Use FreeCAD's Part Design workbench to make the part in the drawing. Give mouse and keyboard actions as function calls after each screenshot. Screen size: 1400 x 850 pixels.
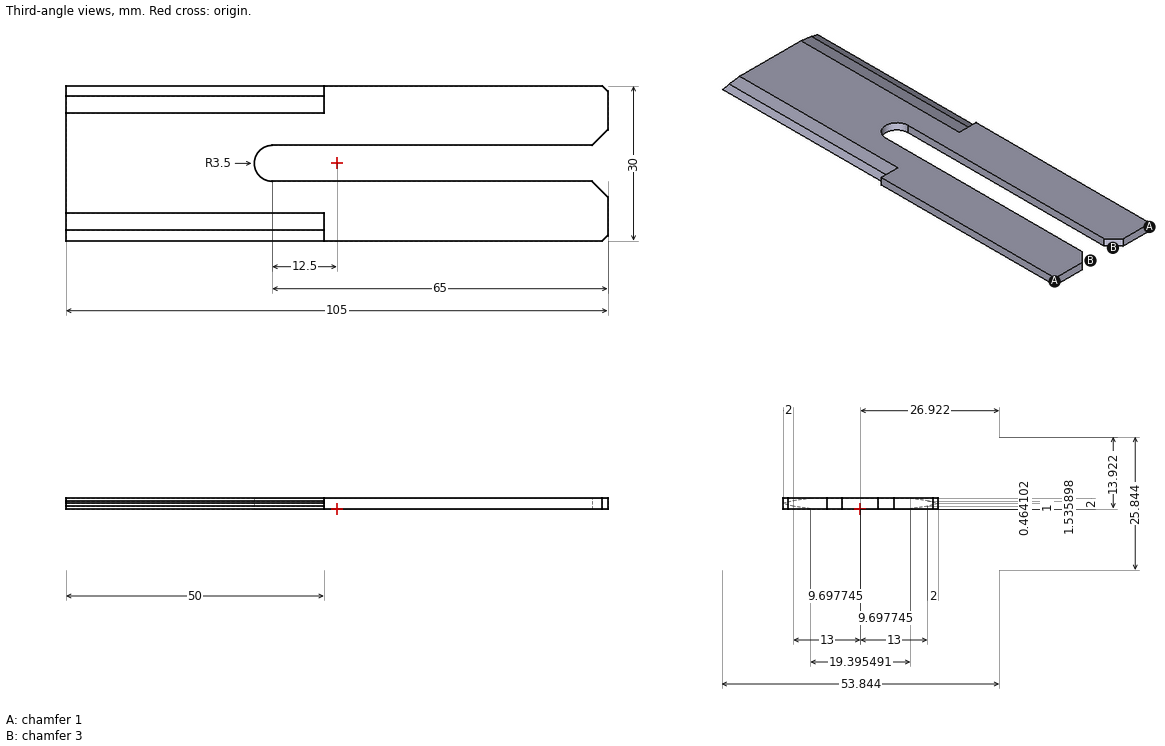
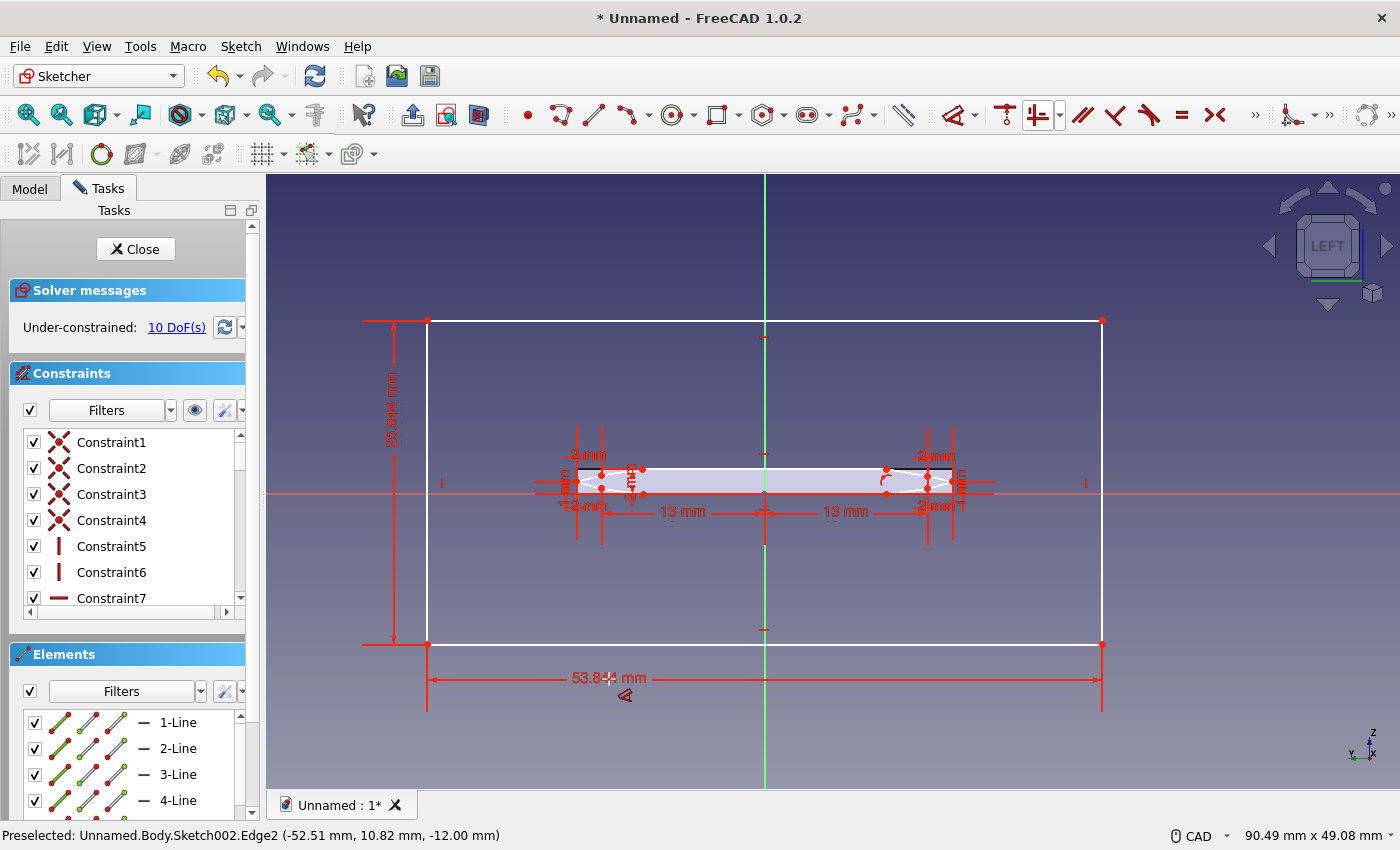
click(427, 321)
click(596, 287)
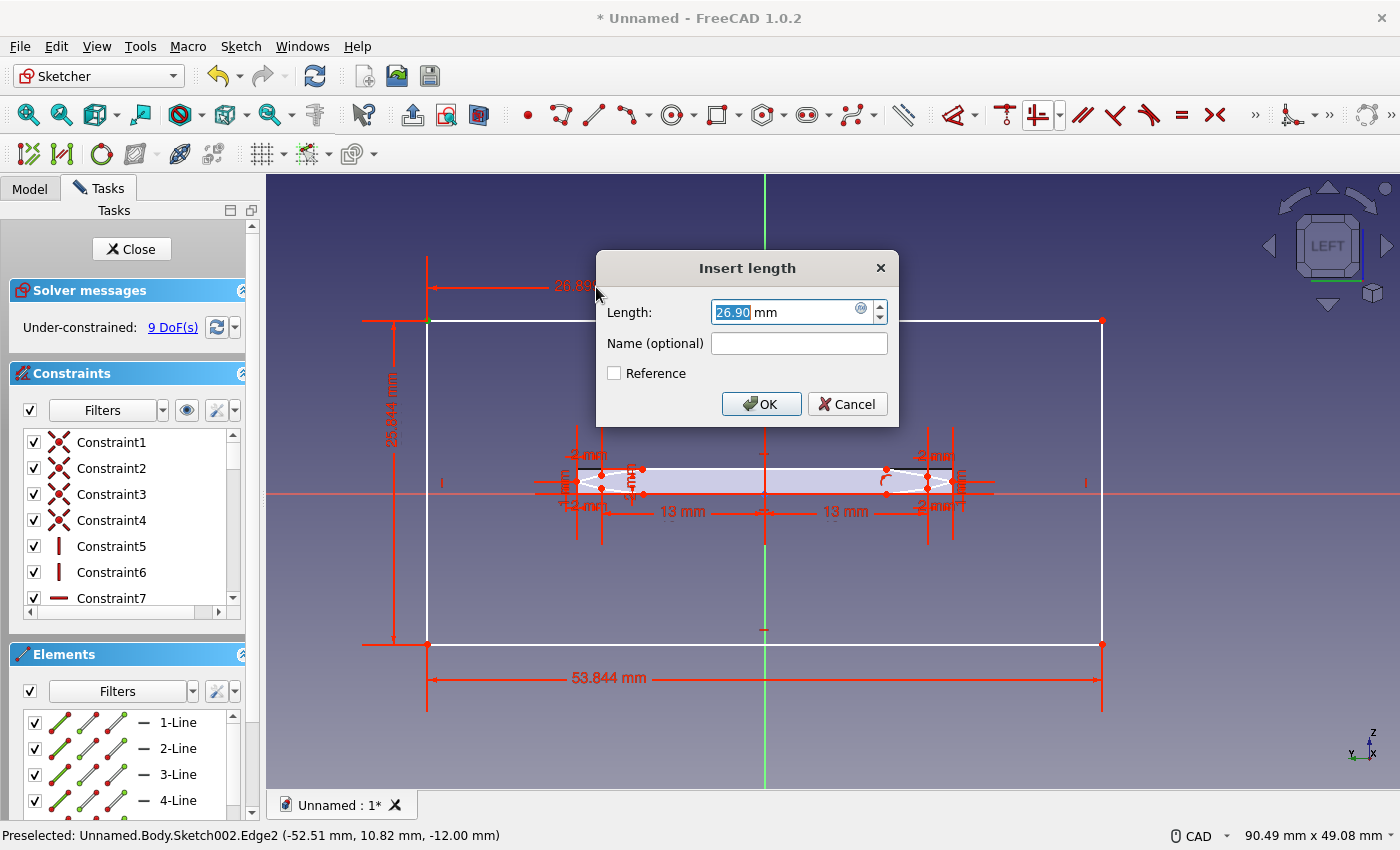
text(26.922)
key(Return)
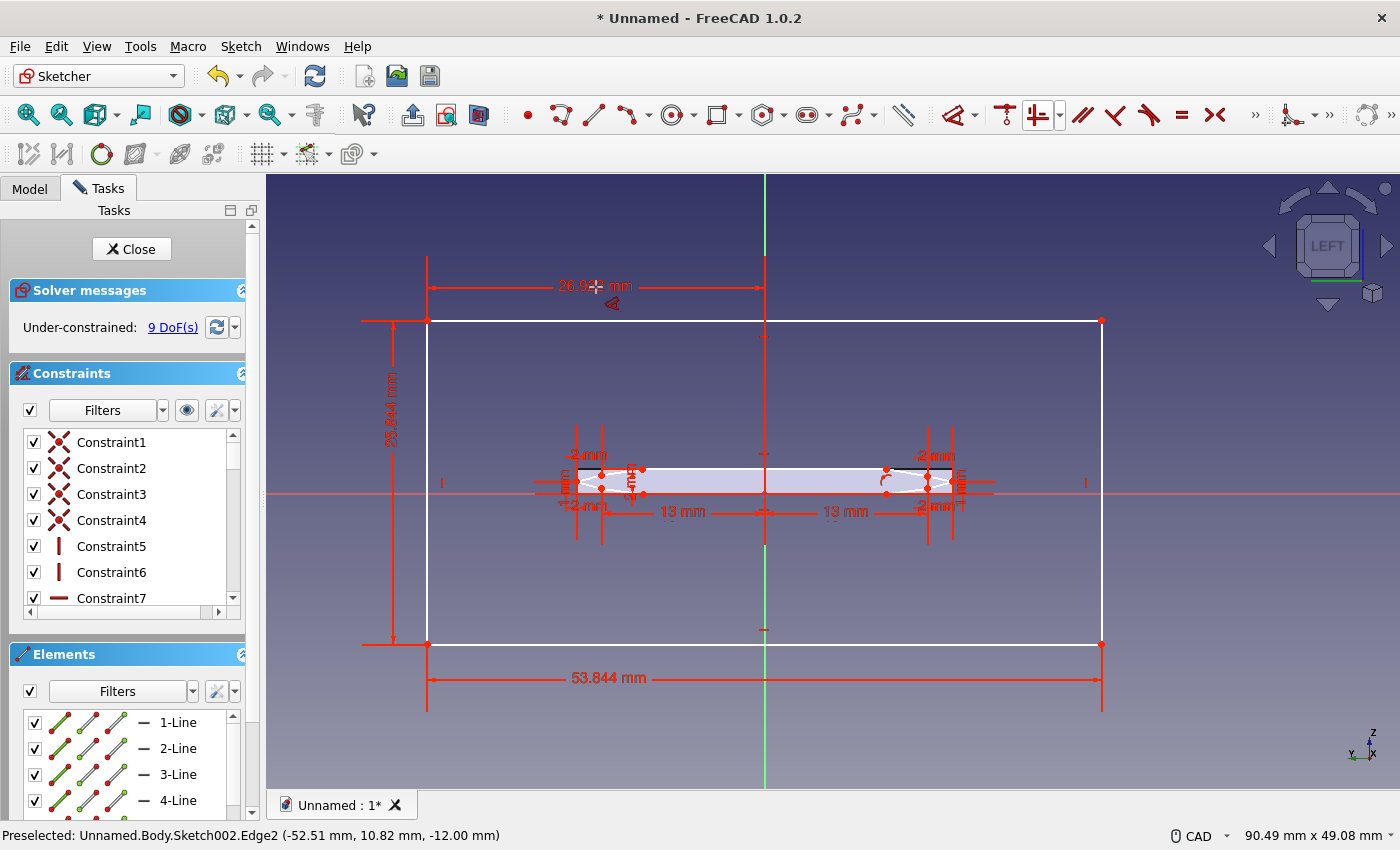
click(427, 321)
click(393, 368)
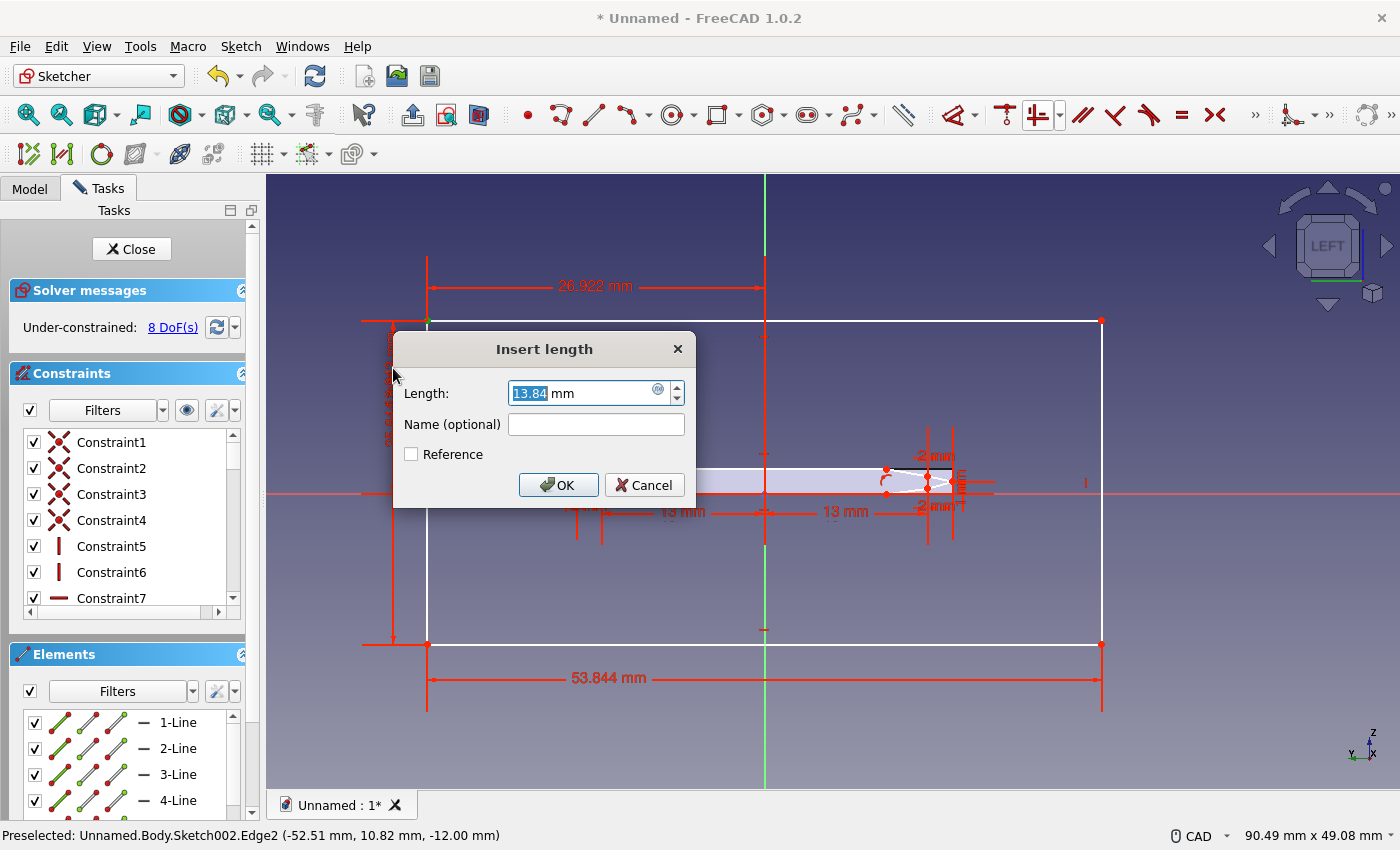
text(13.922)
key(Return)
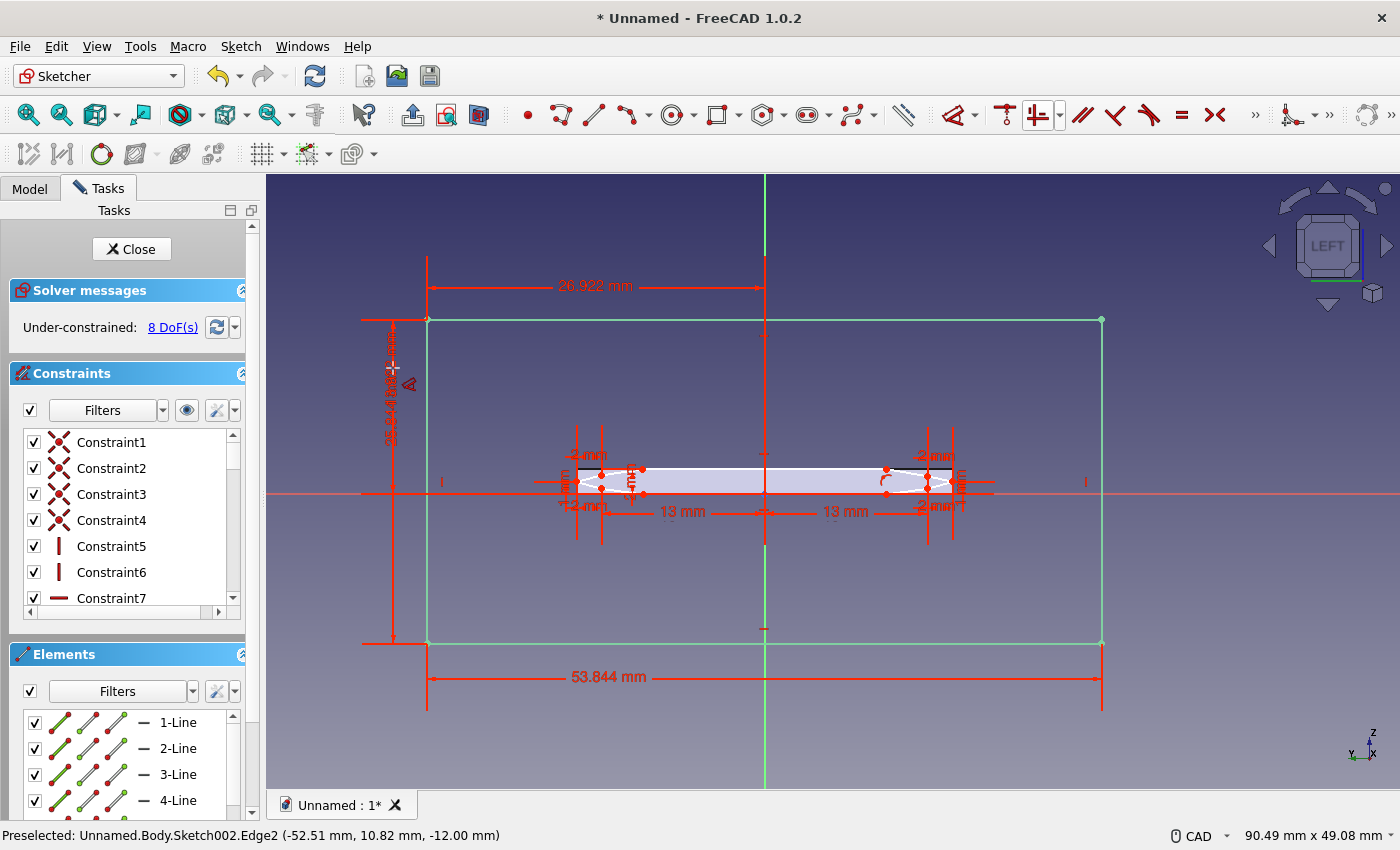
click(813, 494)
click(709, 552)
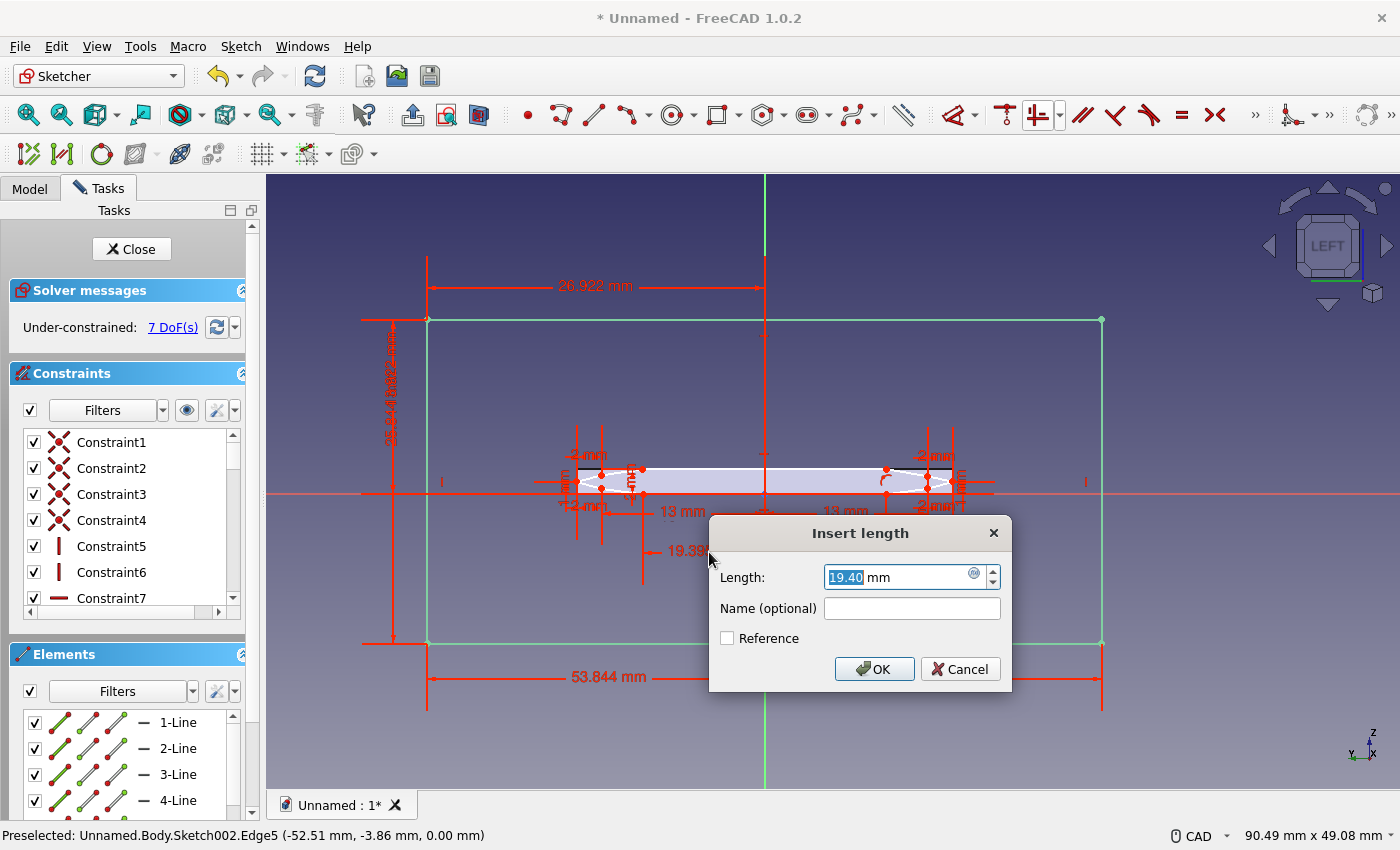
text(19.395491)
key(Return)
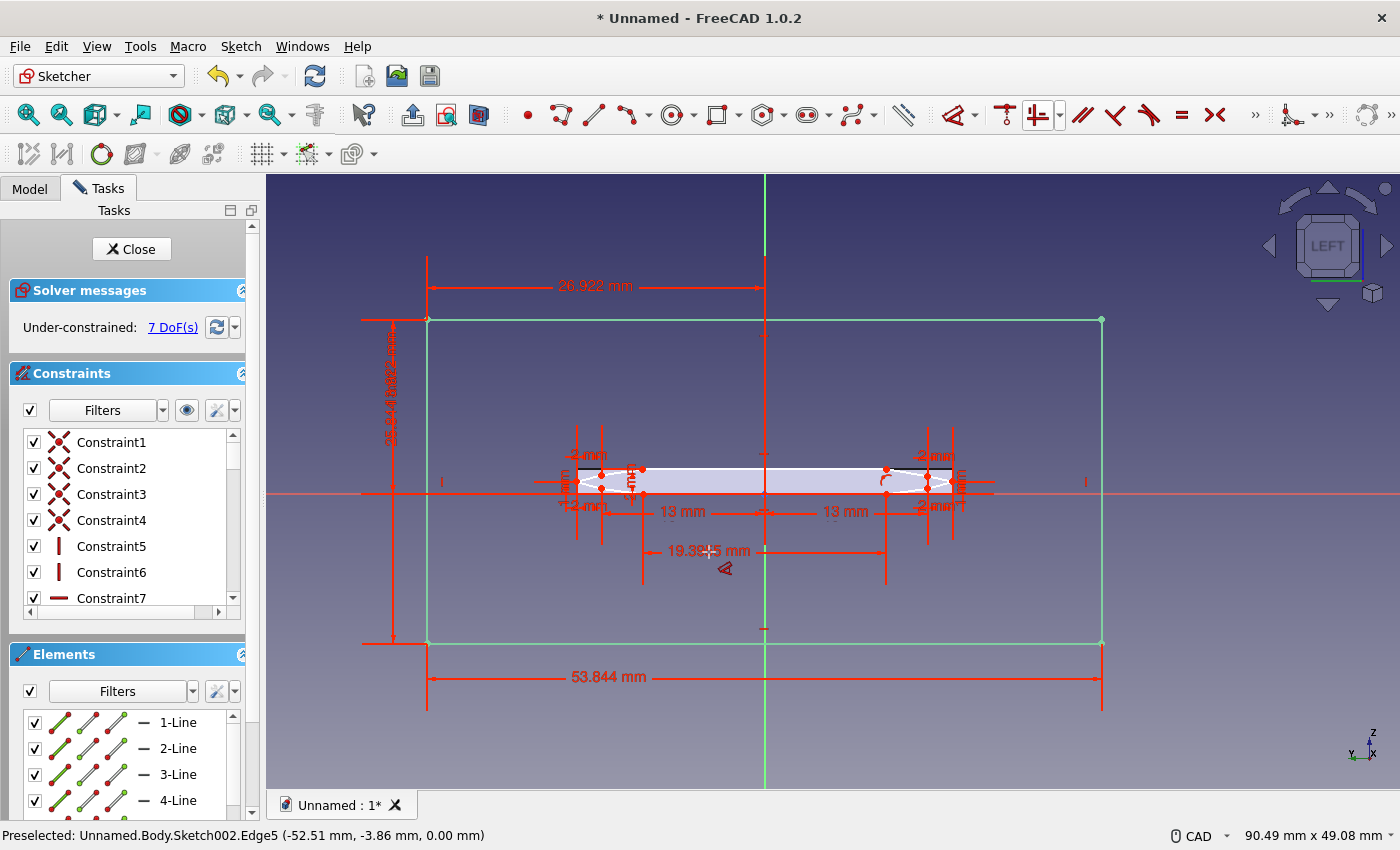
click(716, 469)
click(708, 435)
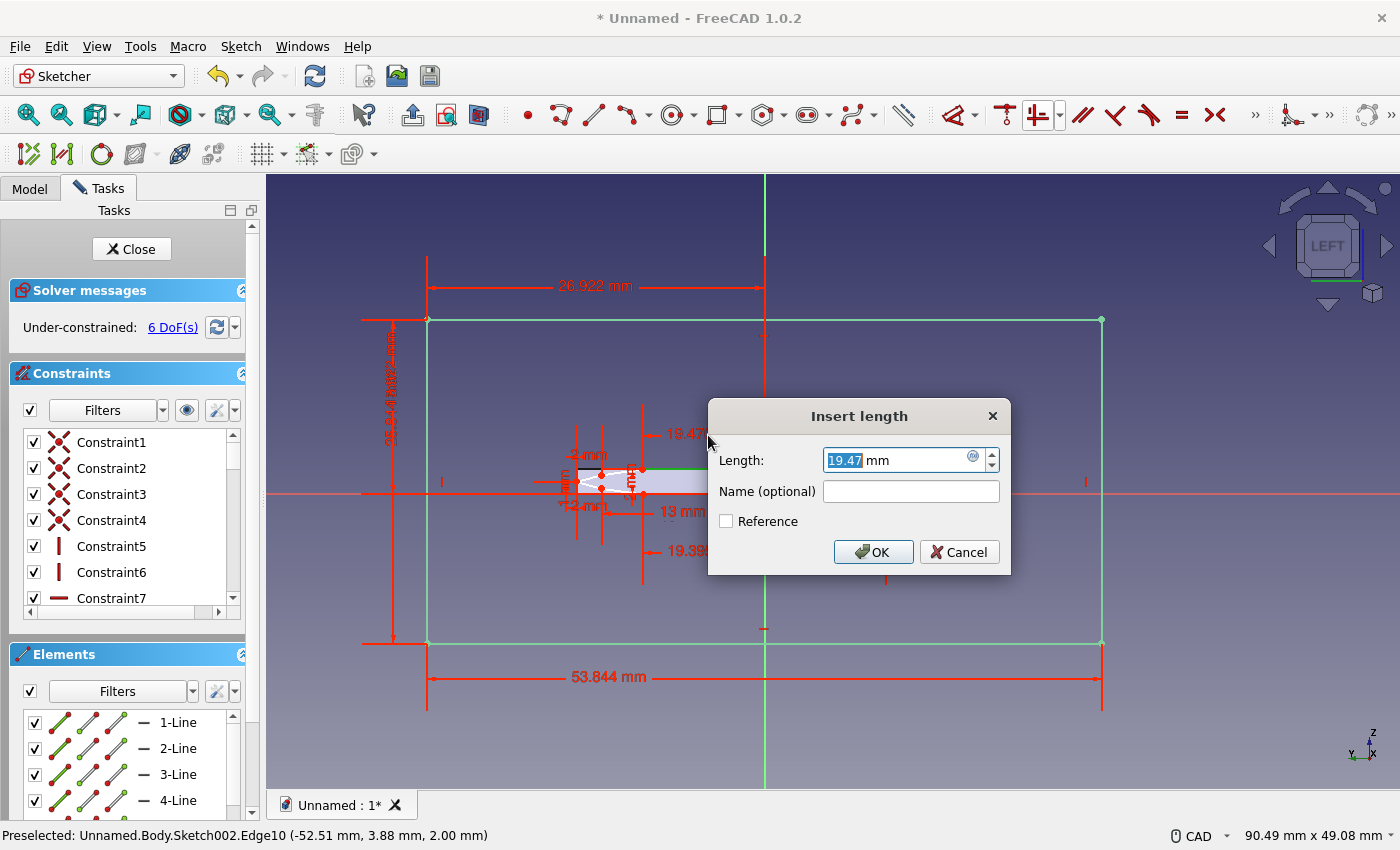
text(19.395491)
key(Return)